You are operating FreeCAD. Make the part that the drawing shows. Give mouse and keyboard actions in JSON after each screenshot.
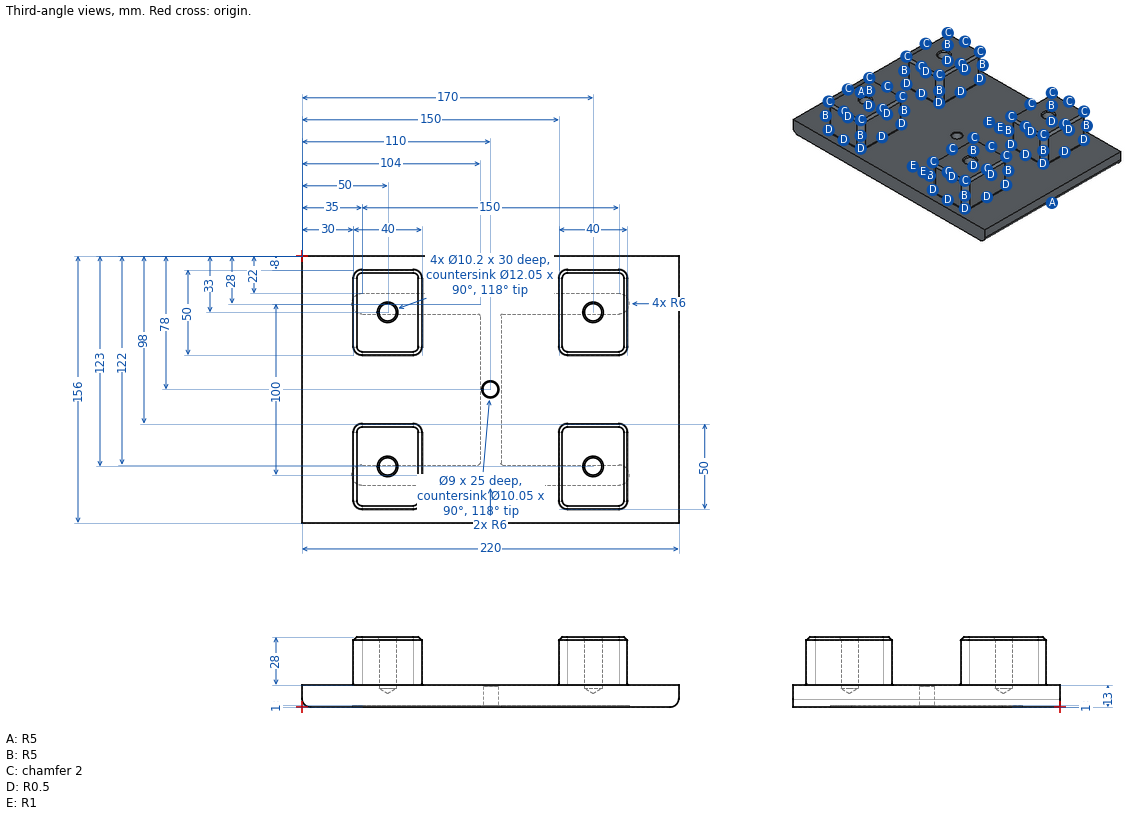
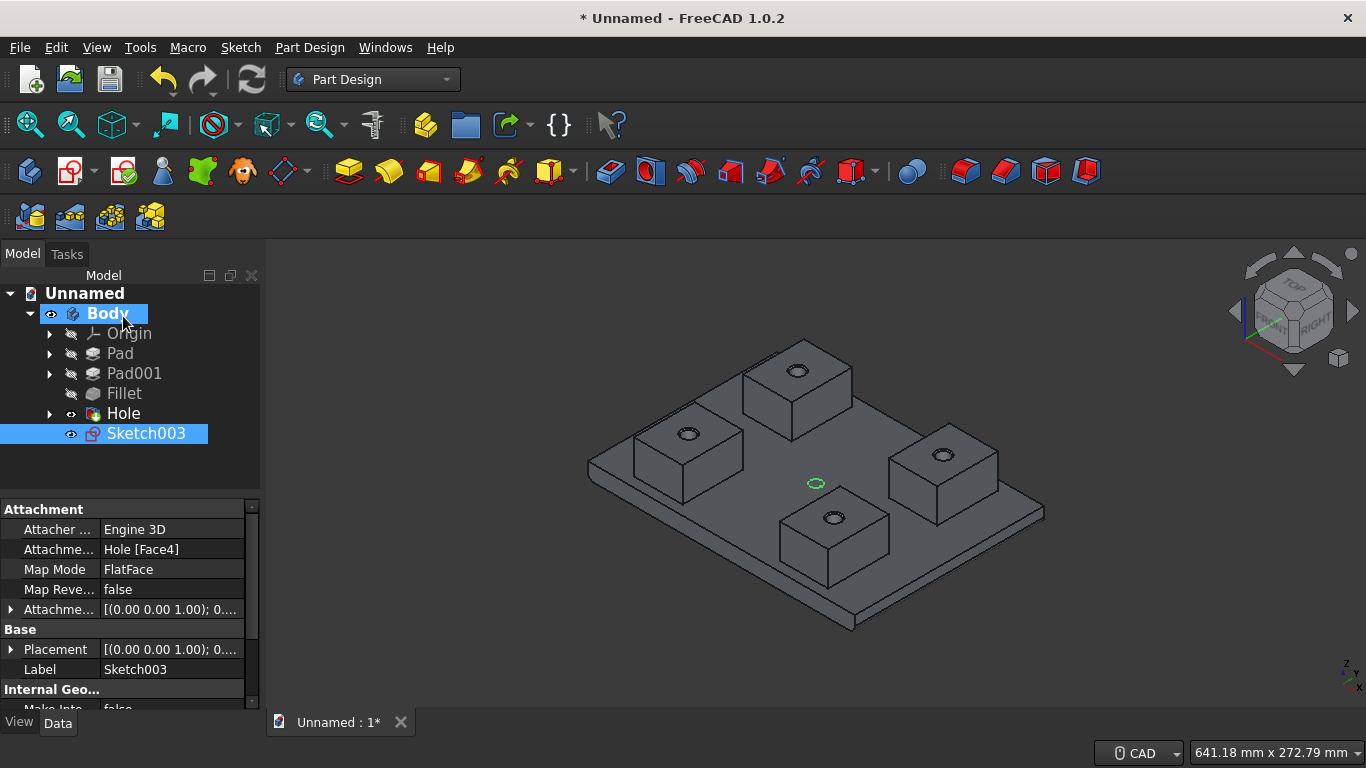
{"action": "left_click", "coordinate": [652, 172]}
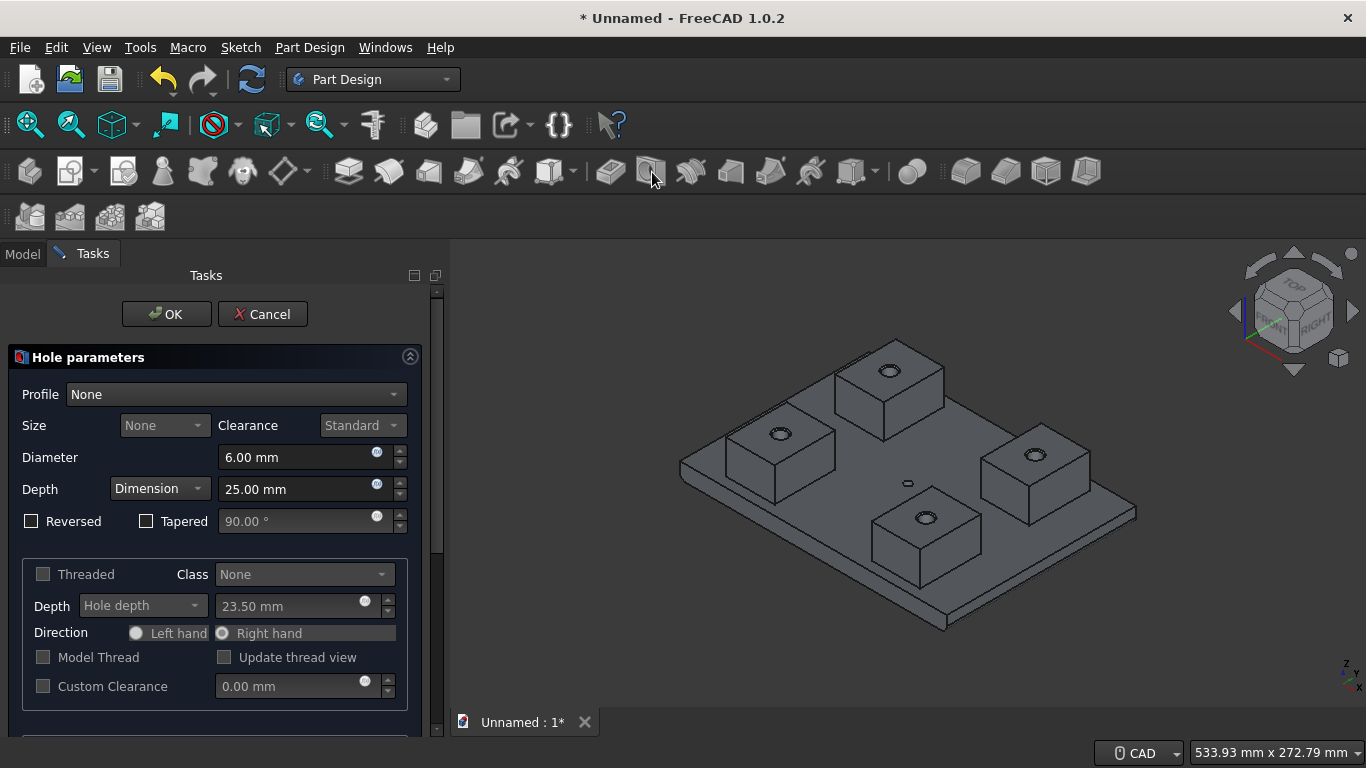
{"action": "triple_click", "coordinate": [305, 457]}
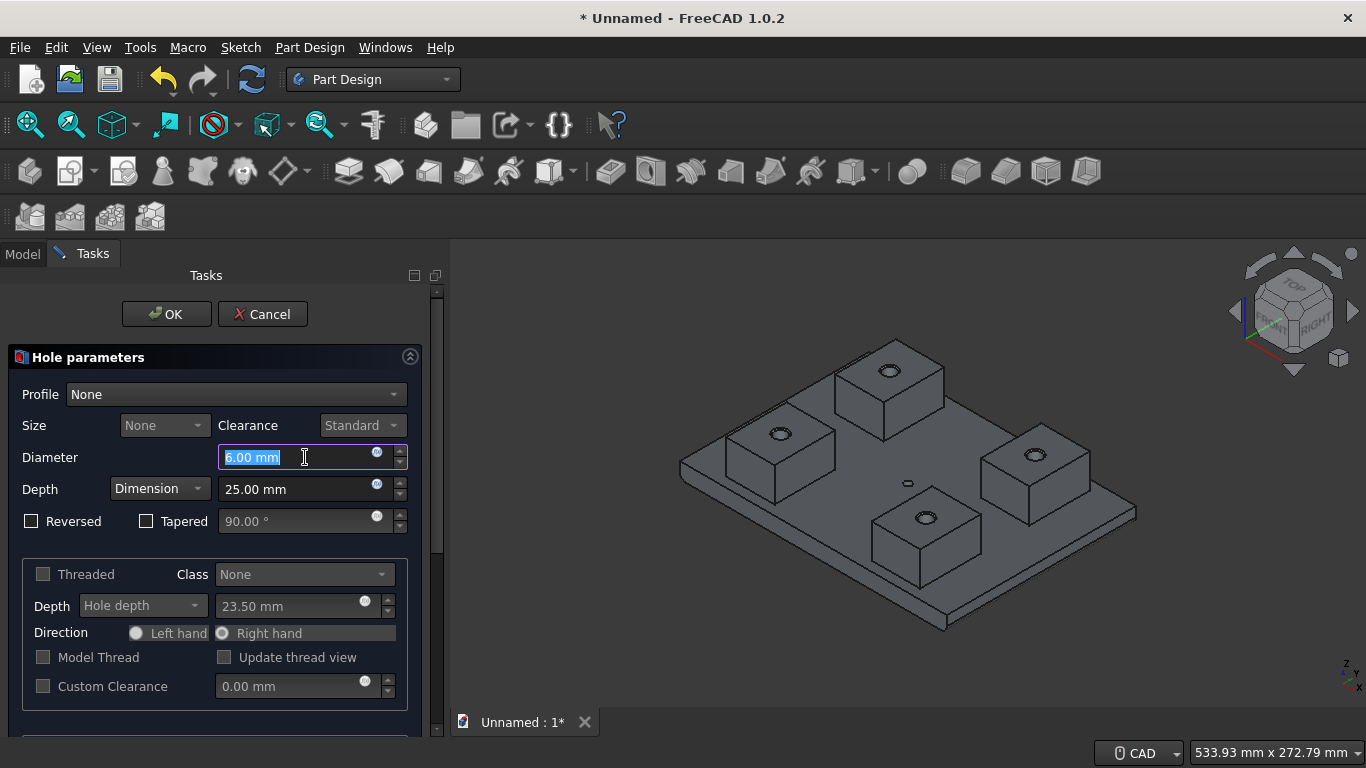
{"action": "type", "text": "9"}
{"action": "key", "text": "Tab"}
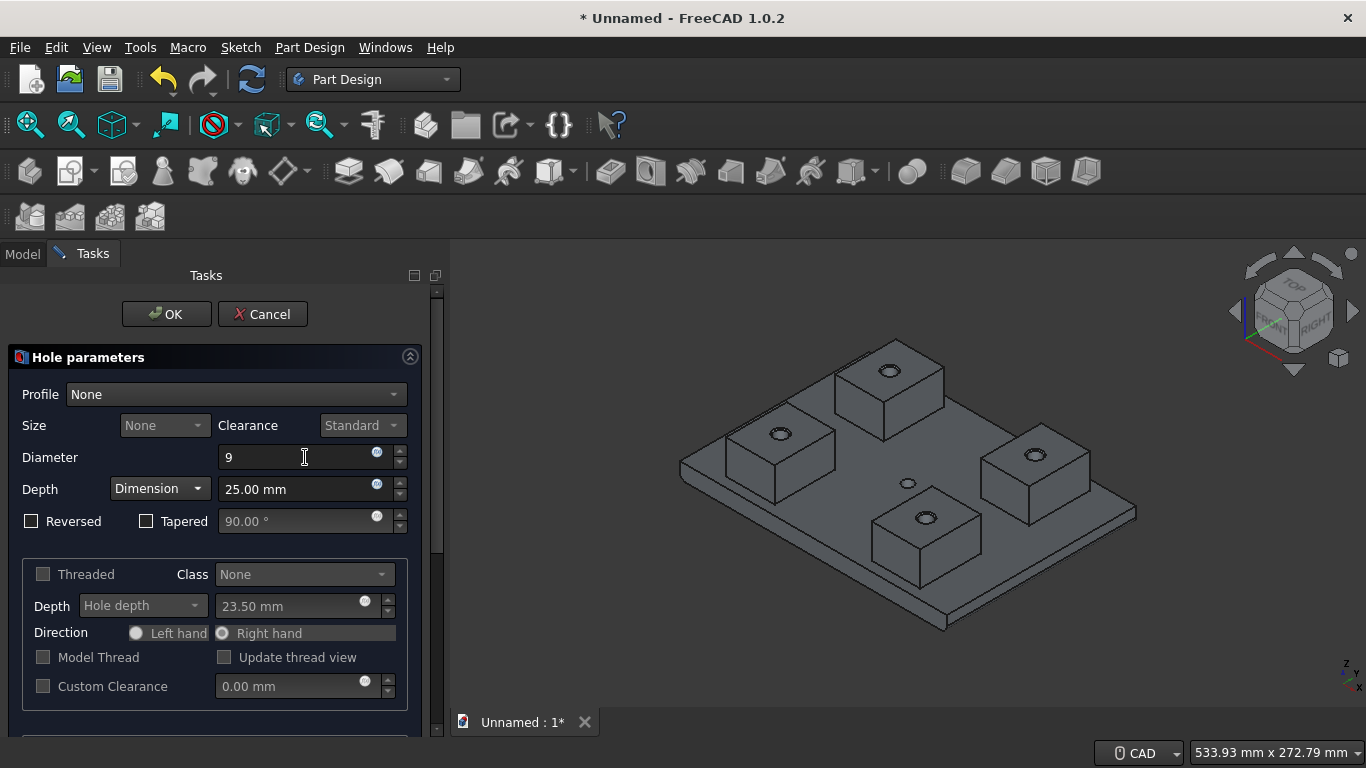
{"action": "triple_click", "coordinate": [305, 489]}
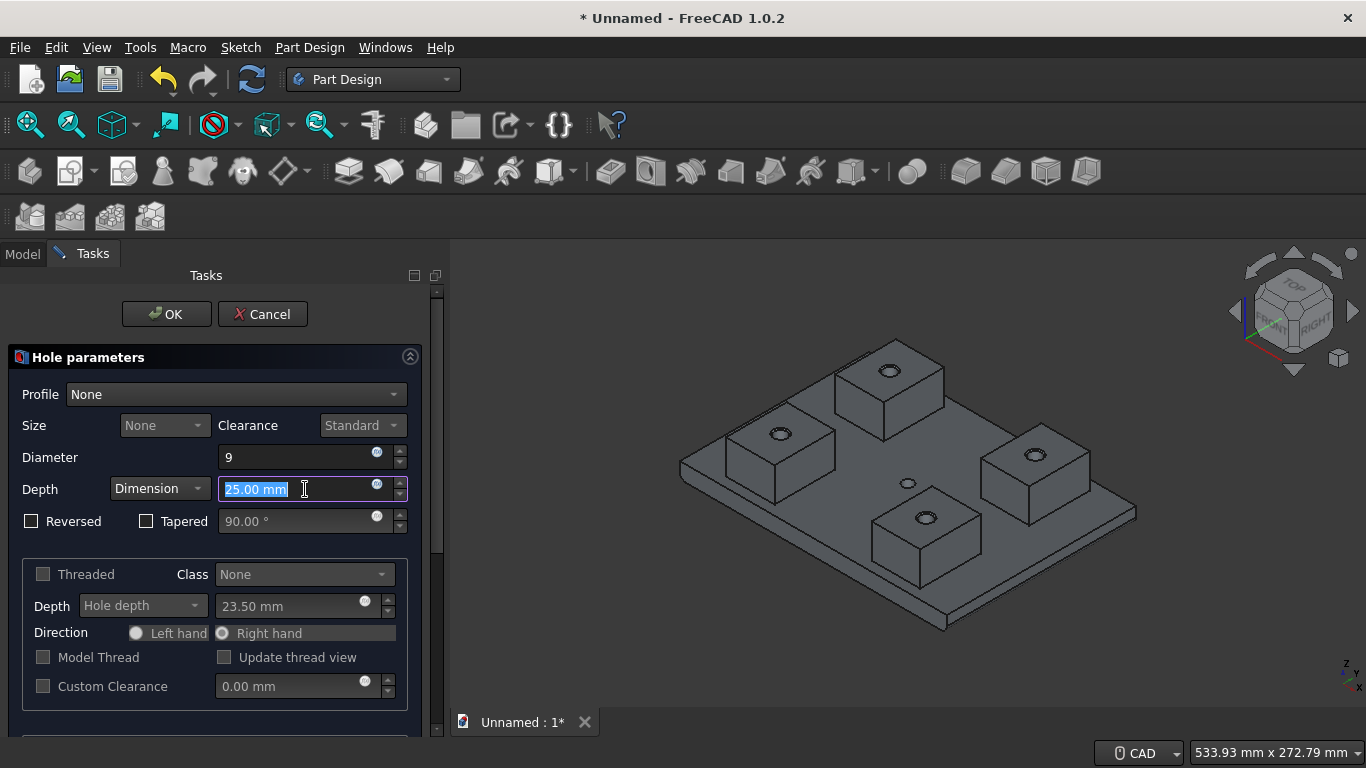
{"action": "type", "text": "25"}
{"action": "key", "text": "Tab"}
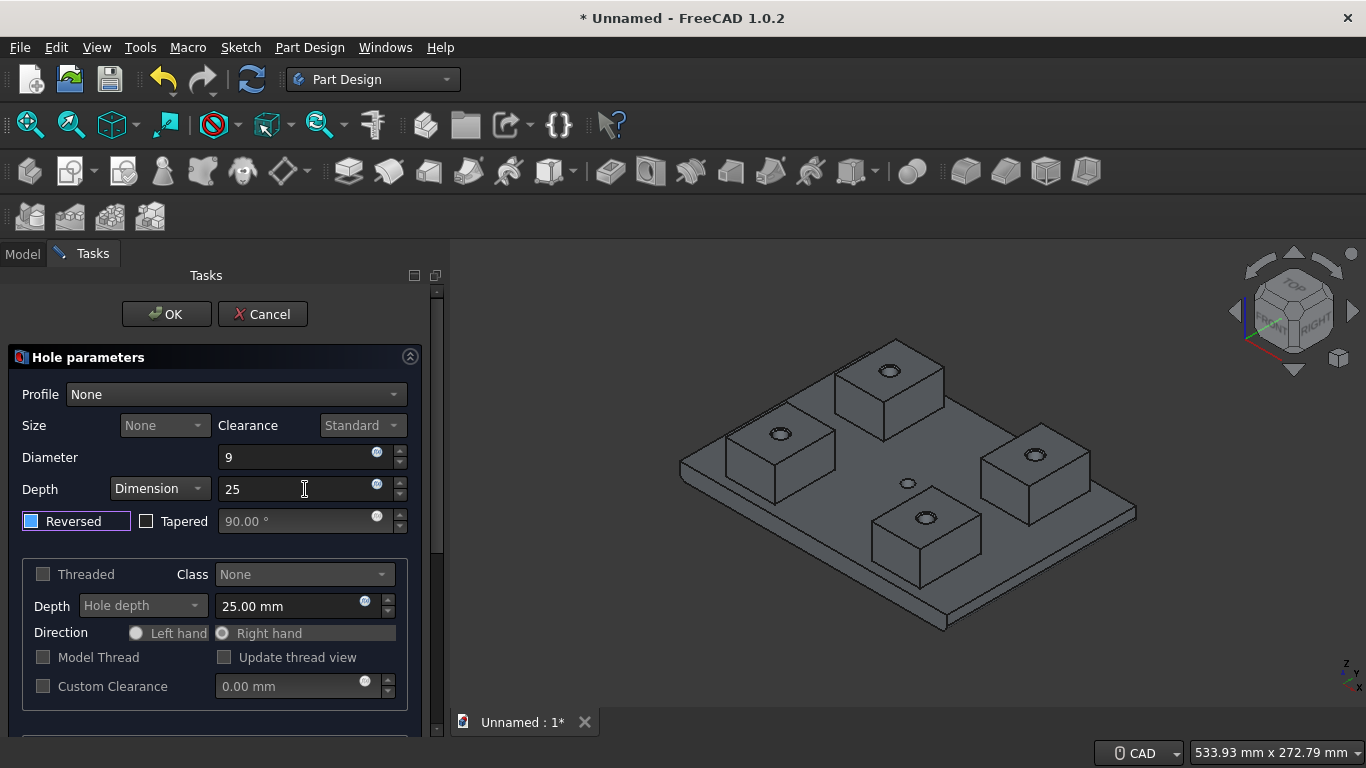
{"action": "scroll", "coordinate": [437, 510], "scroll_direction": "down", "scroll_amount": 2}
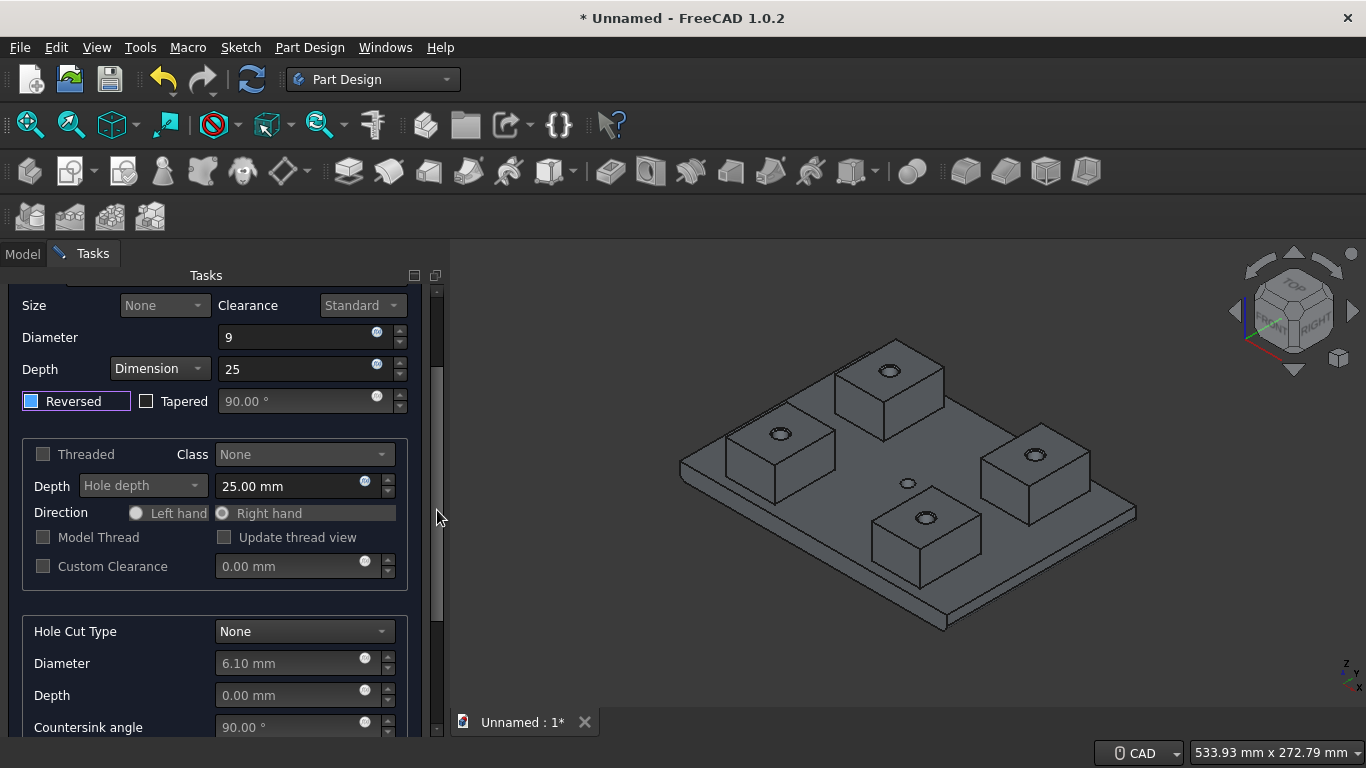
{"action": "left_click", "coordinate": [306, 632]}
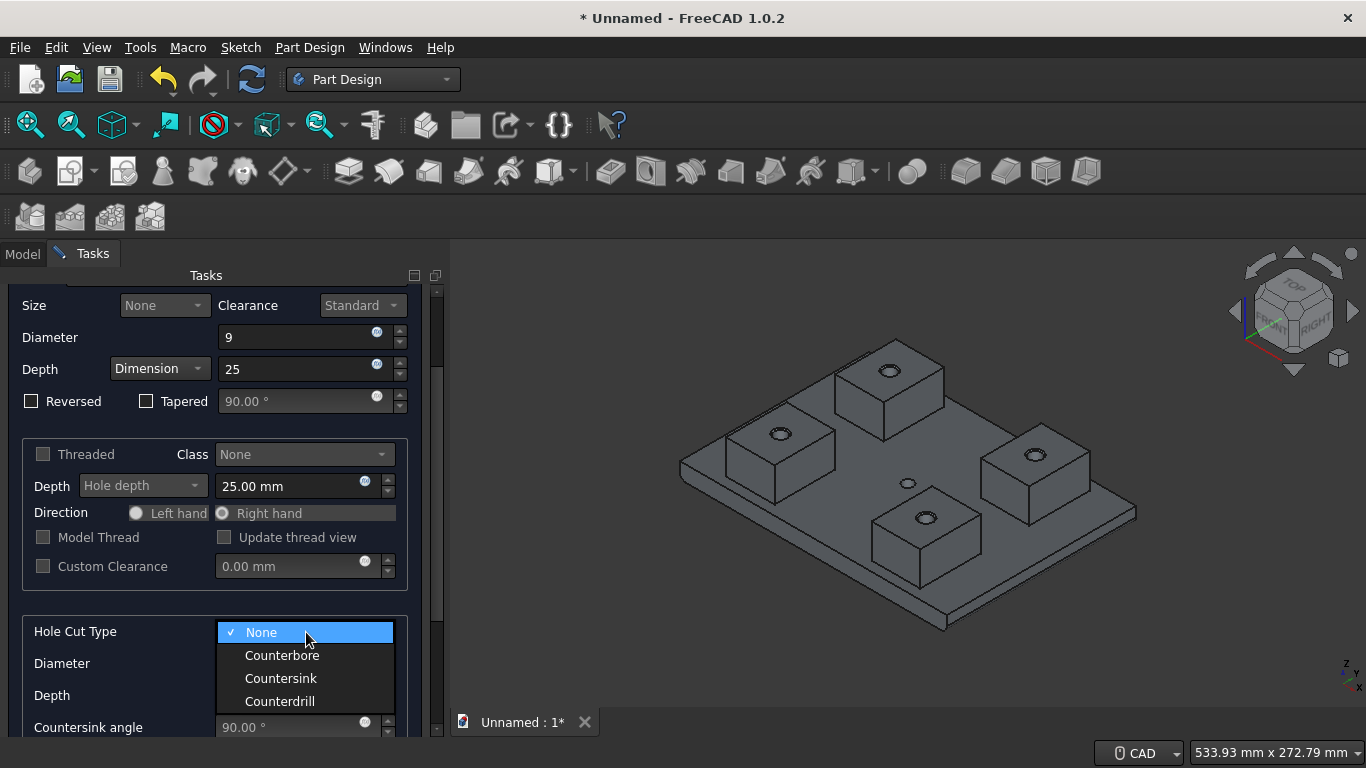
{"action": "left_click", "coordinate": [304, 678]}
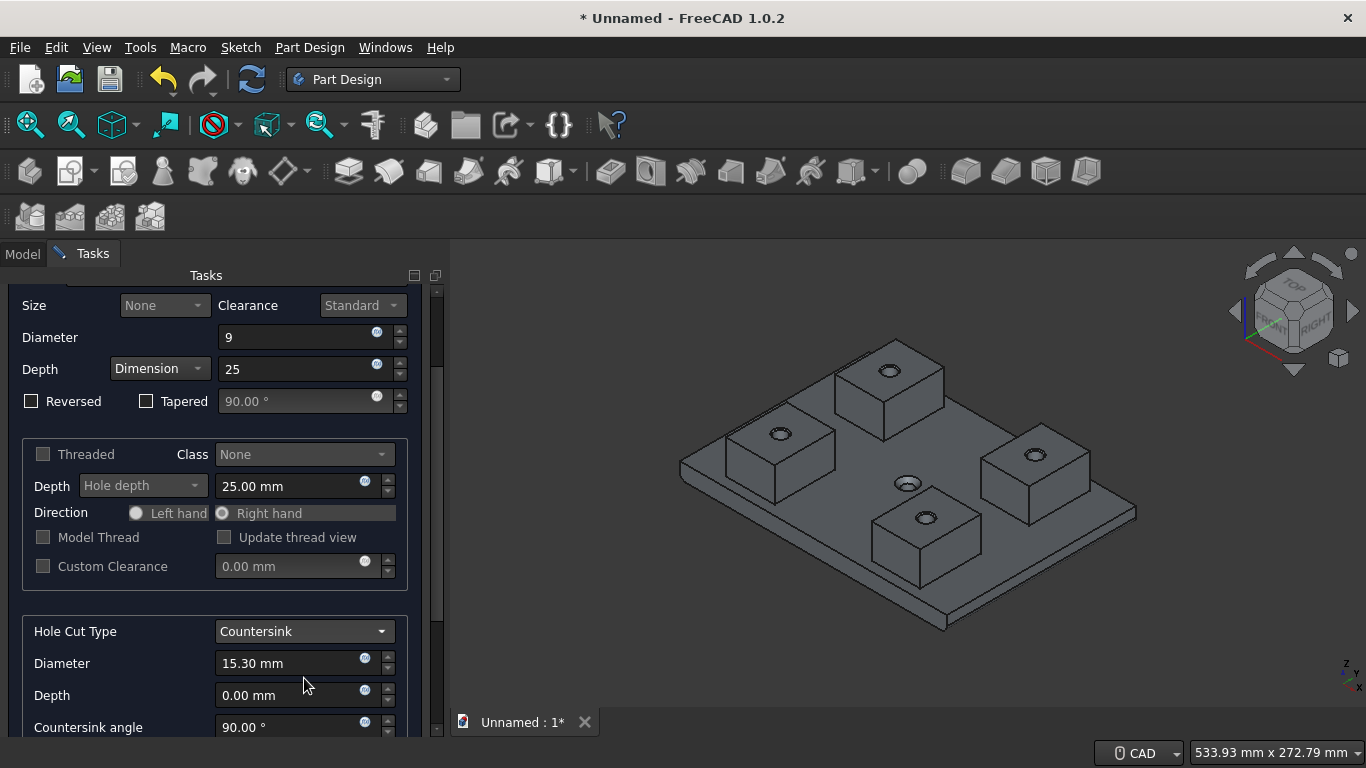
{"action": "triple_click", "coordinate": [298, 663]}